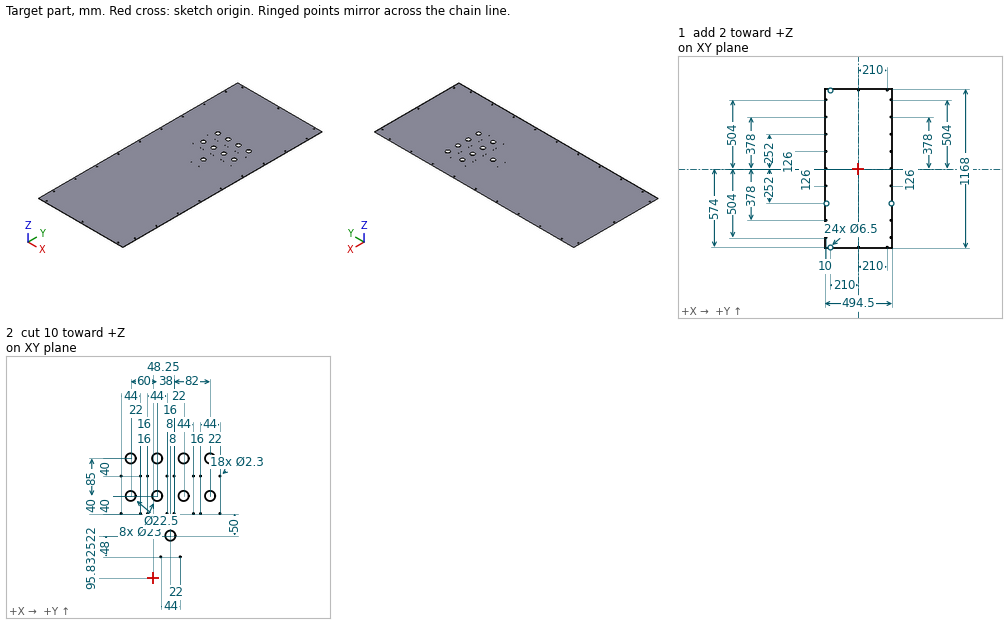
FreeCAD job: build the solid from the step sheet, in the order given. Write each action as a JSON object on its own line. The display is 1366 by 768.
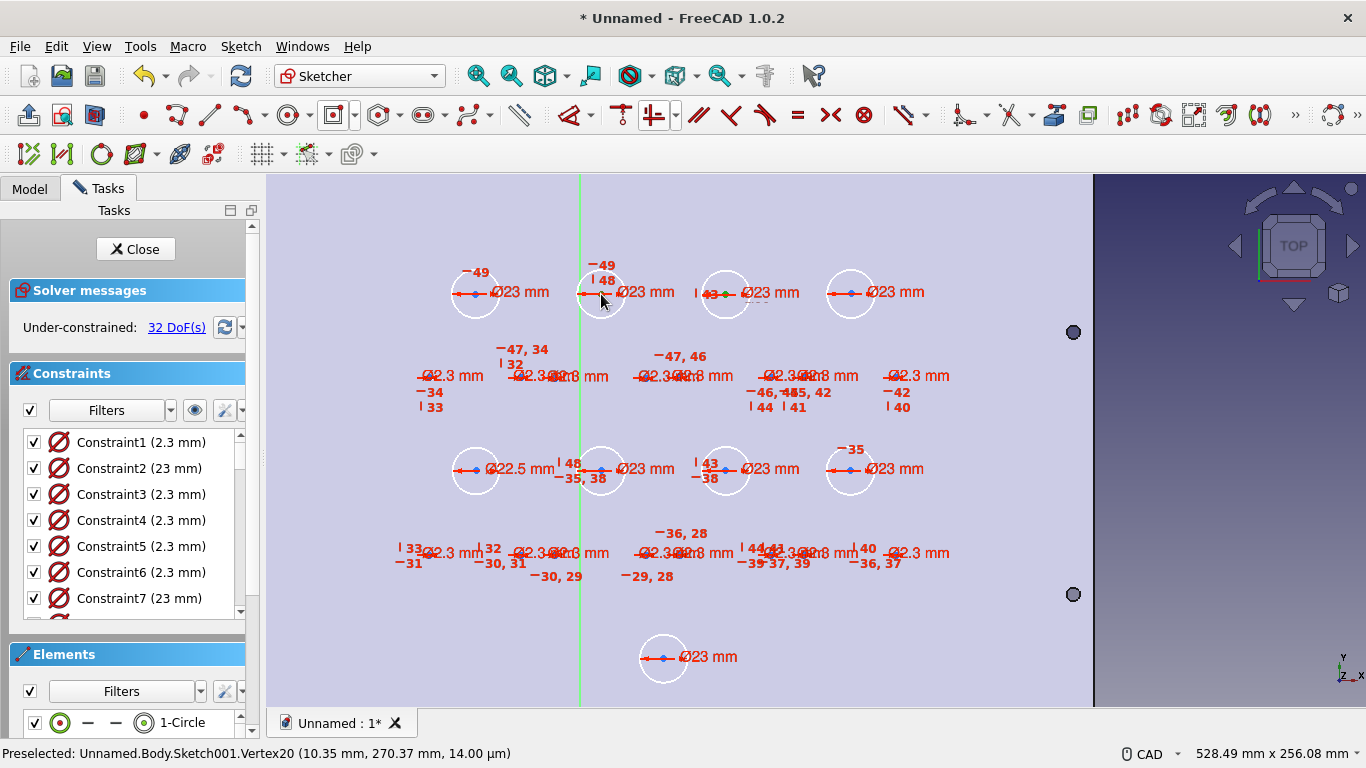
{"action": "key", "text": "h"}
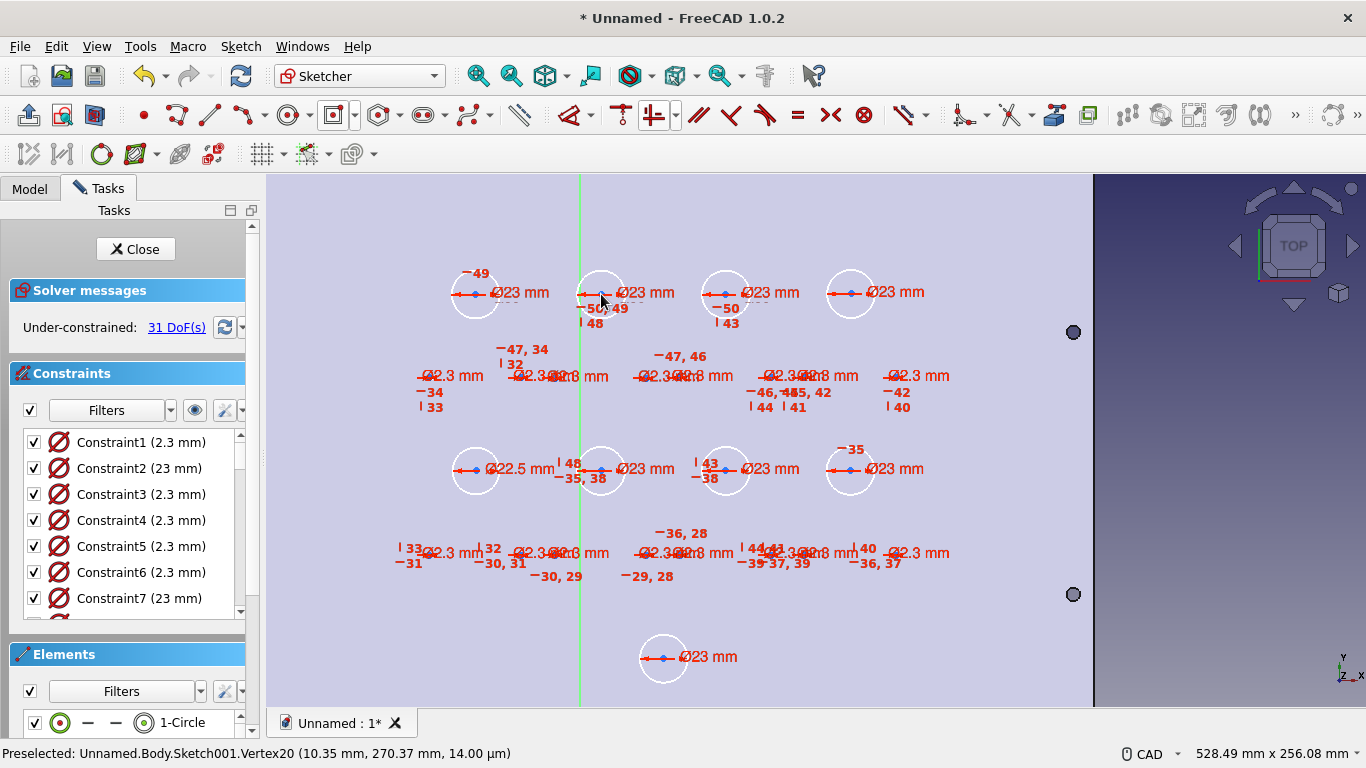
{"action": "left_click", "coordinate": [680, 378]}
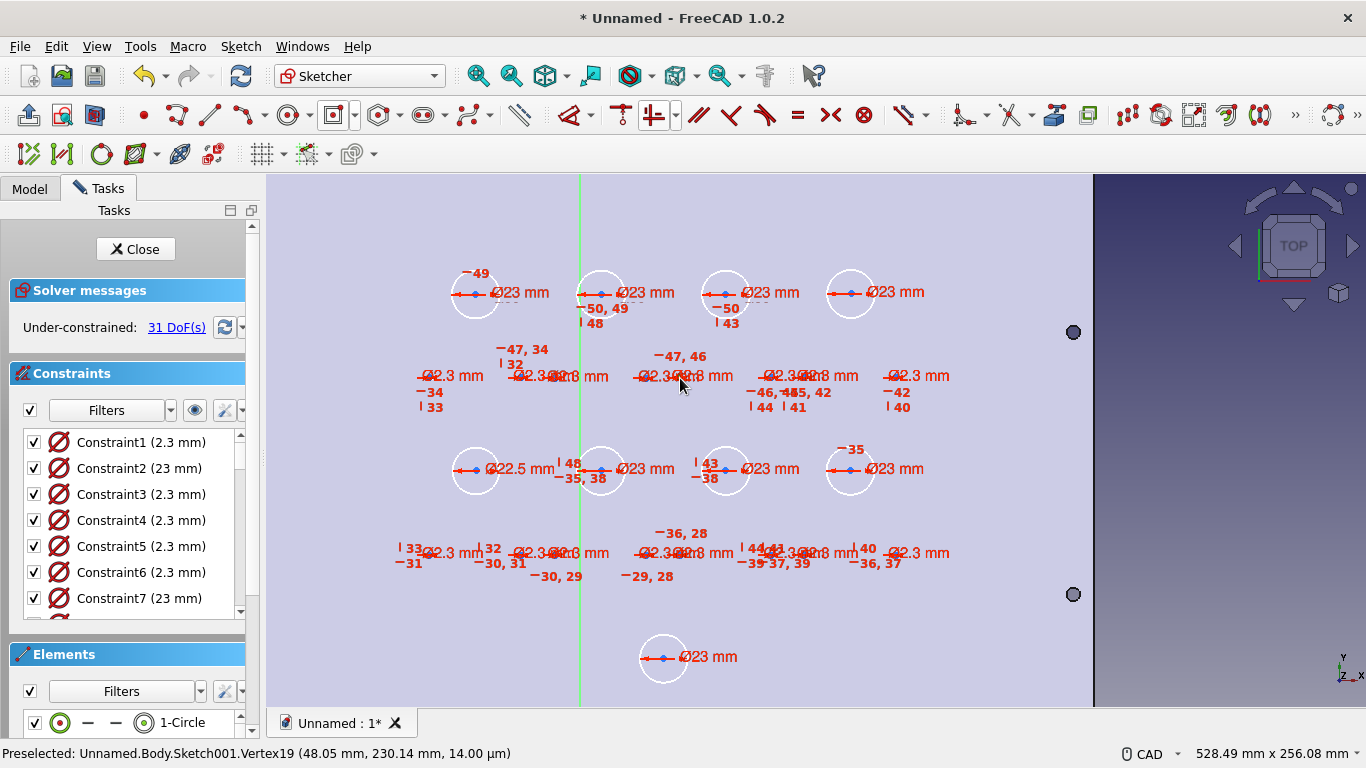
{"action": "left_click", "coordinate": [646, 378]}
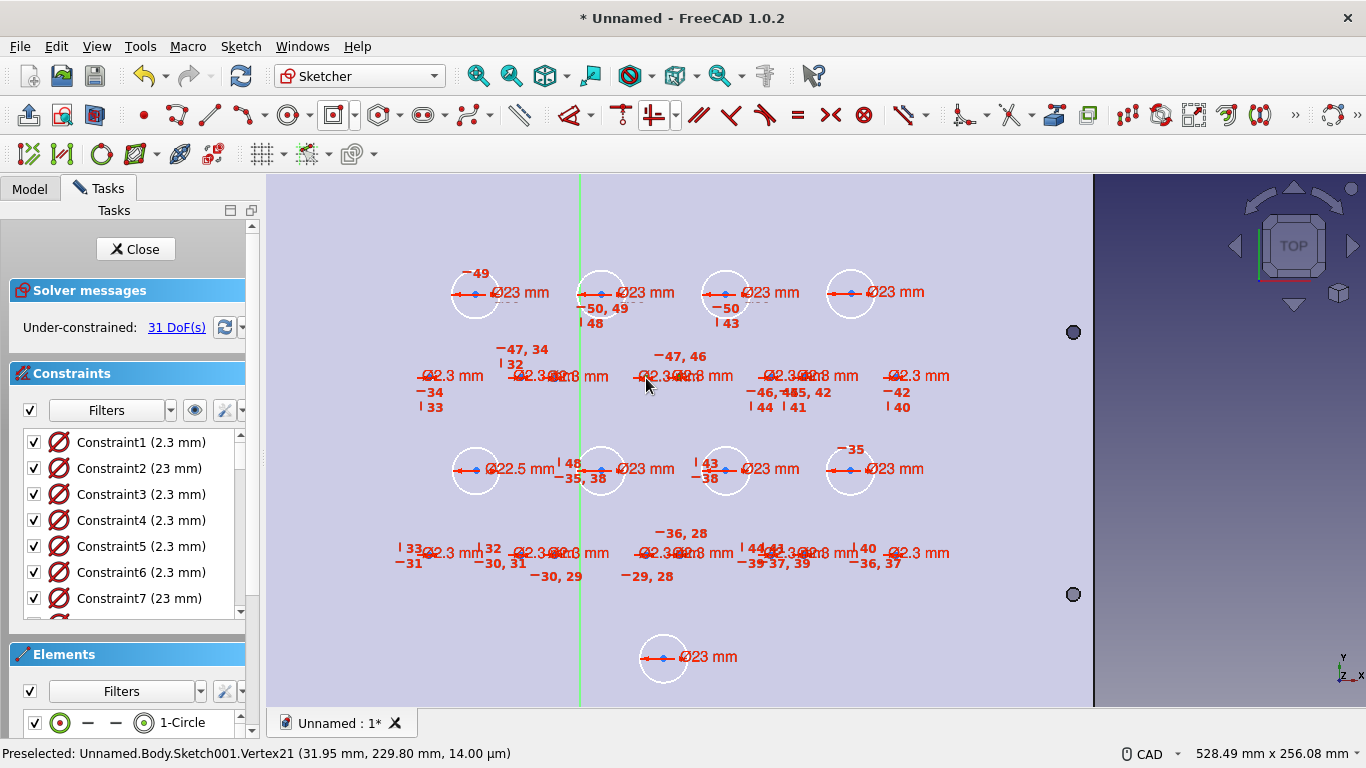
{"action": "left_click", "coordinate": [676, 116]}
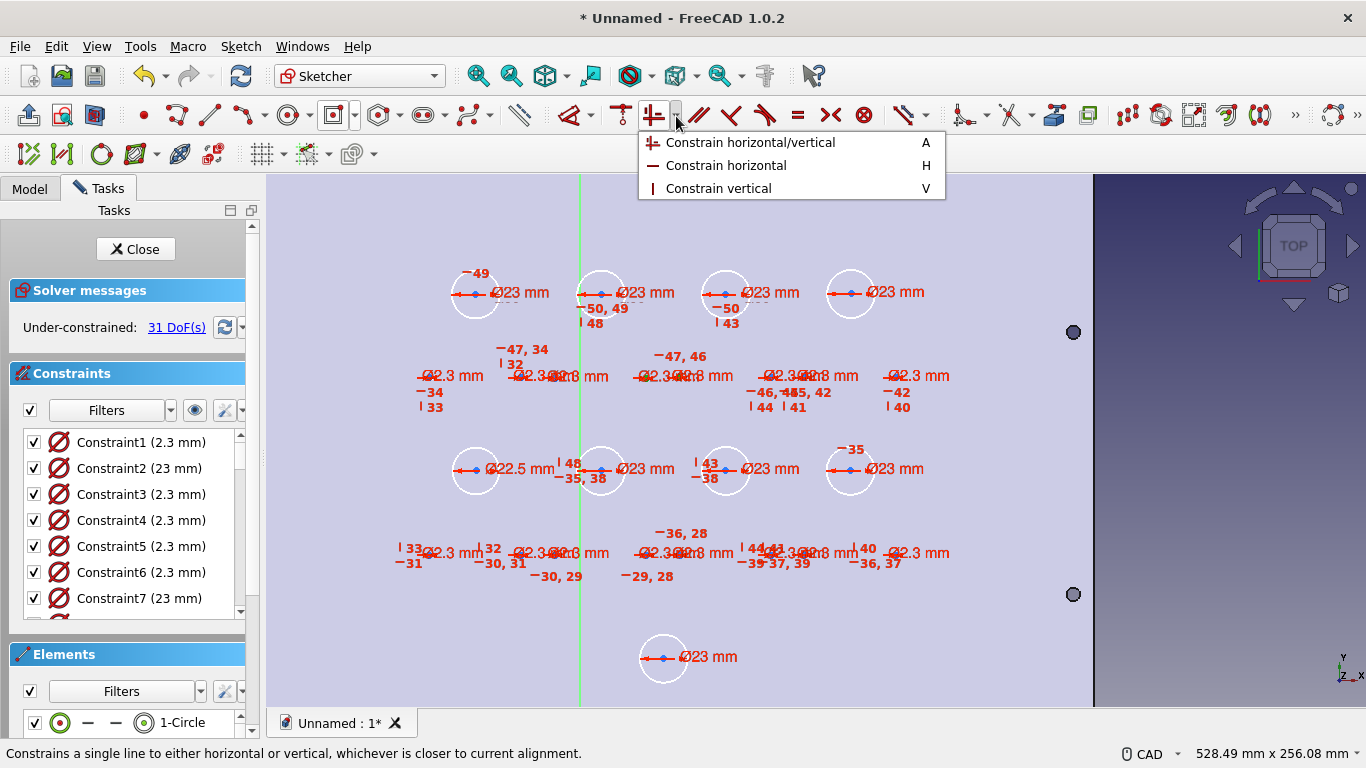
{"action": "left_click", "coordinate": [792, 166]}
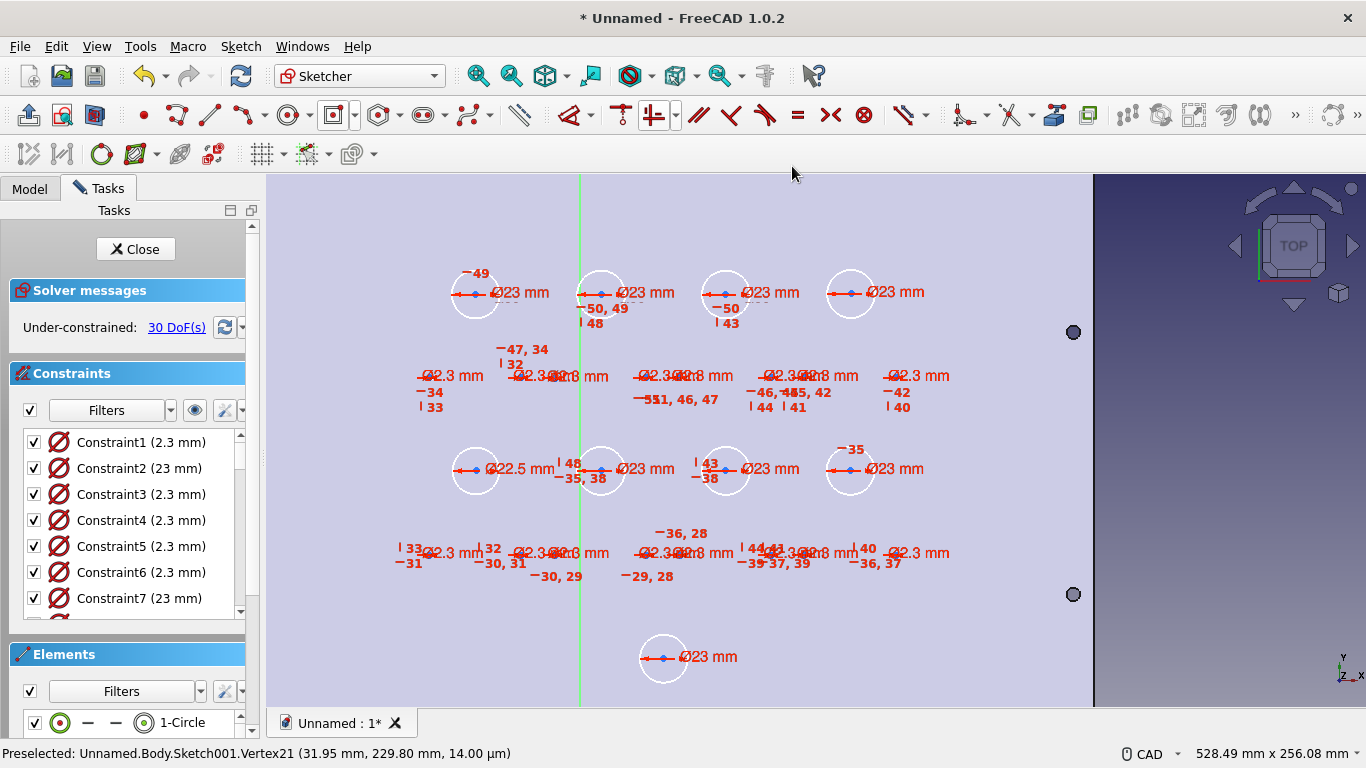
{"action": "left_click", "coordinate": [521, 378]}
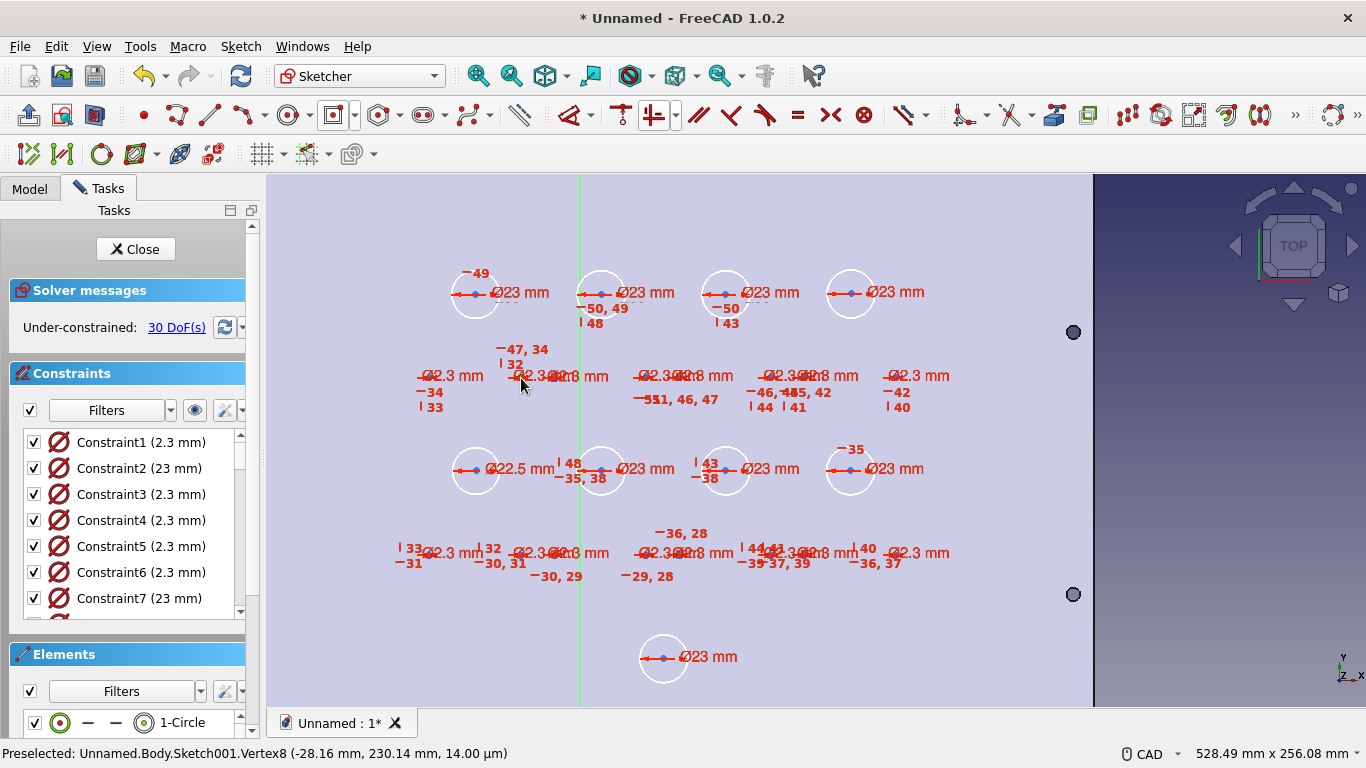
{"action": "left_click", "coordinate": [555, 378]}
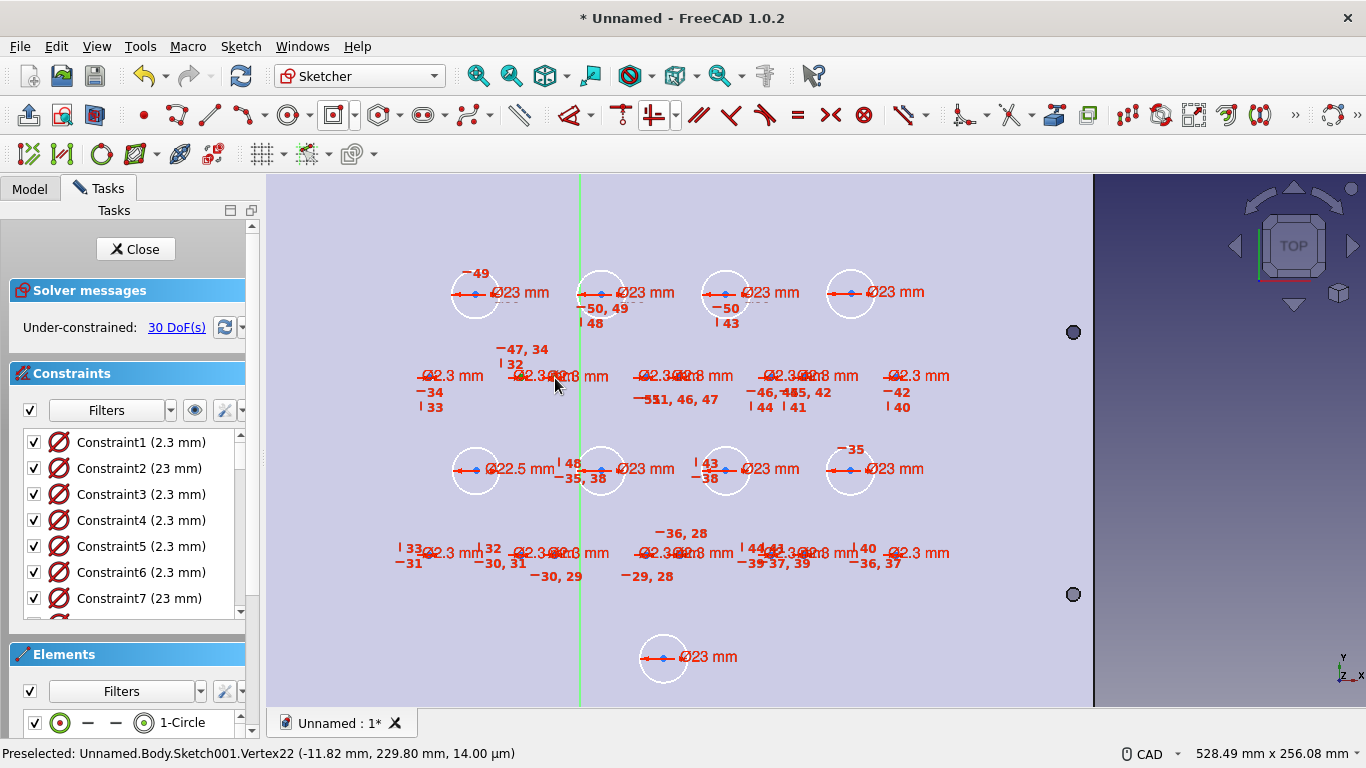
{"action": "left_click", "coordinate": [676, 116]}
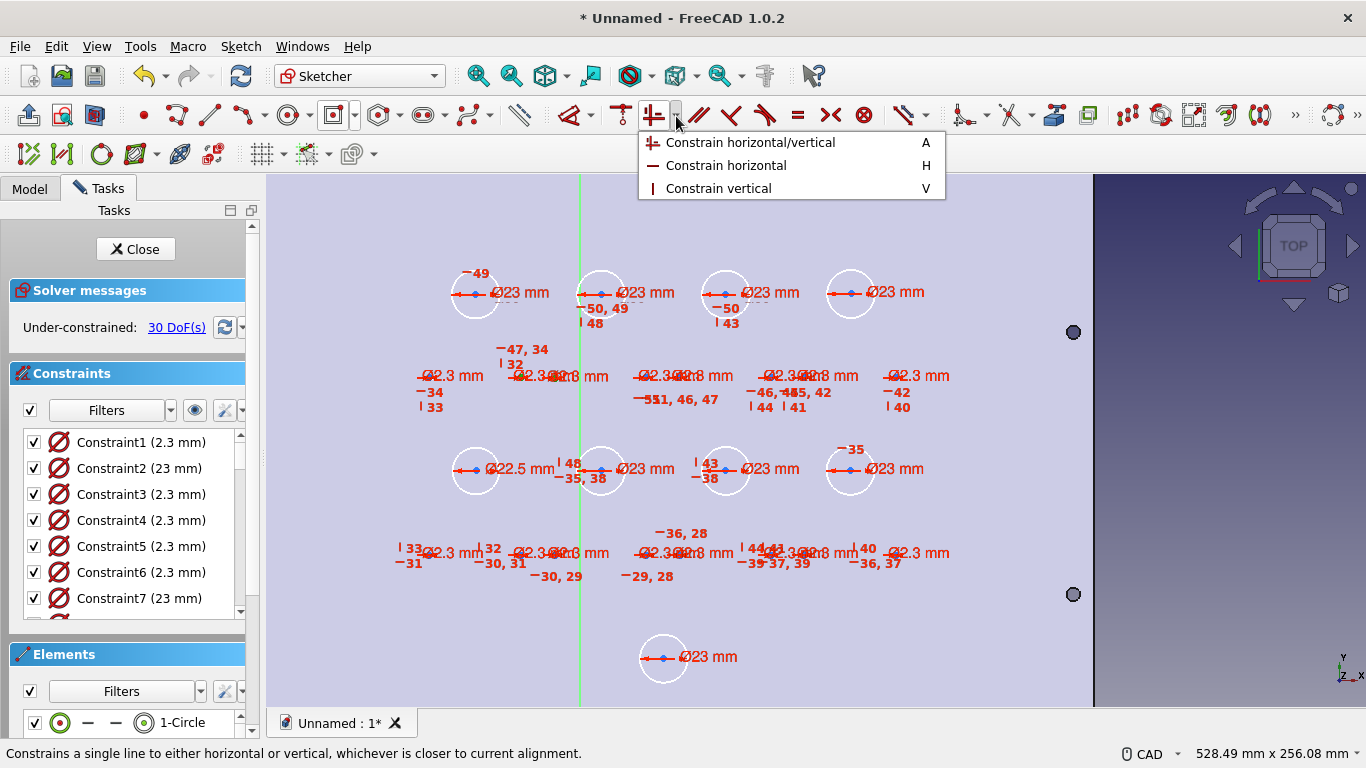
{"action": "left_click", "coordinate": [792, 166]}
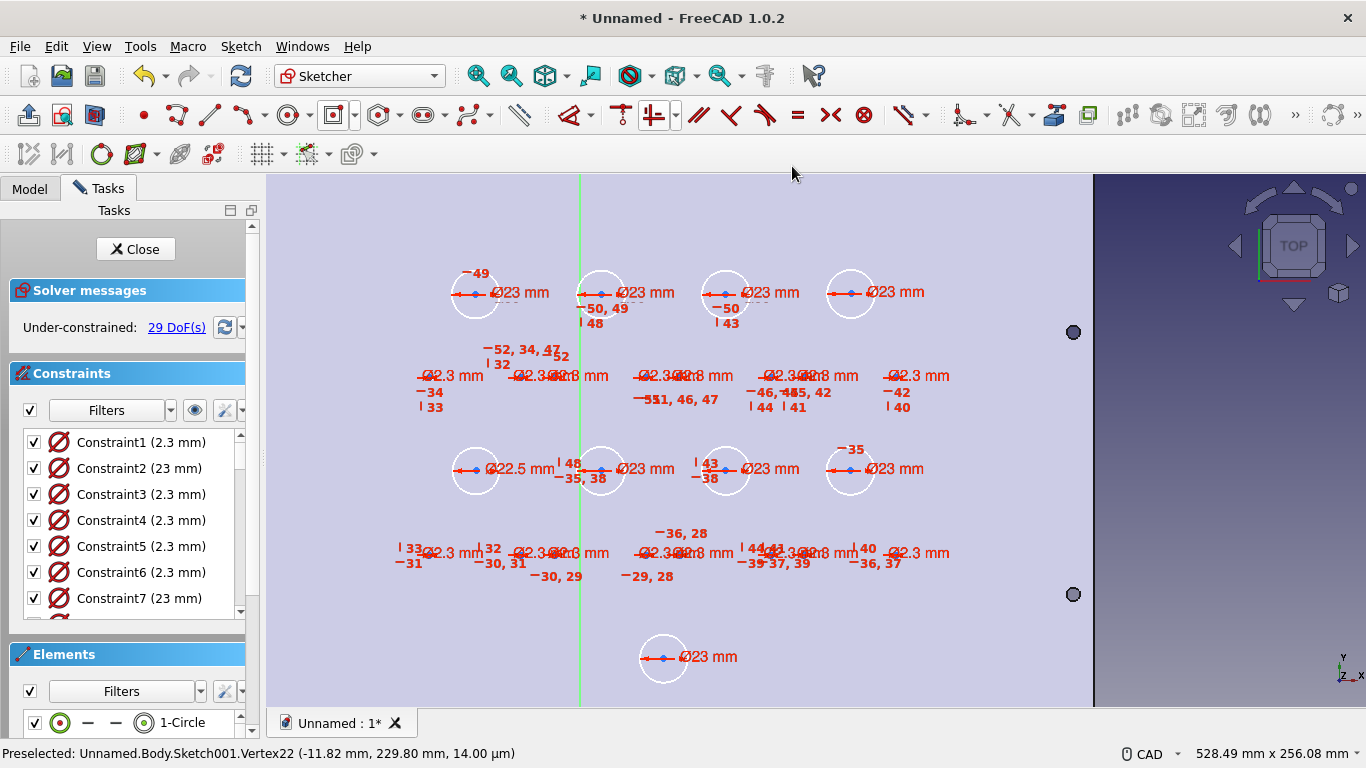
{"action": "scroll", "coordinate": [850, 292], "scroll_direction": "down", "scroll_amount": 3}